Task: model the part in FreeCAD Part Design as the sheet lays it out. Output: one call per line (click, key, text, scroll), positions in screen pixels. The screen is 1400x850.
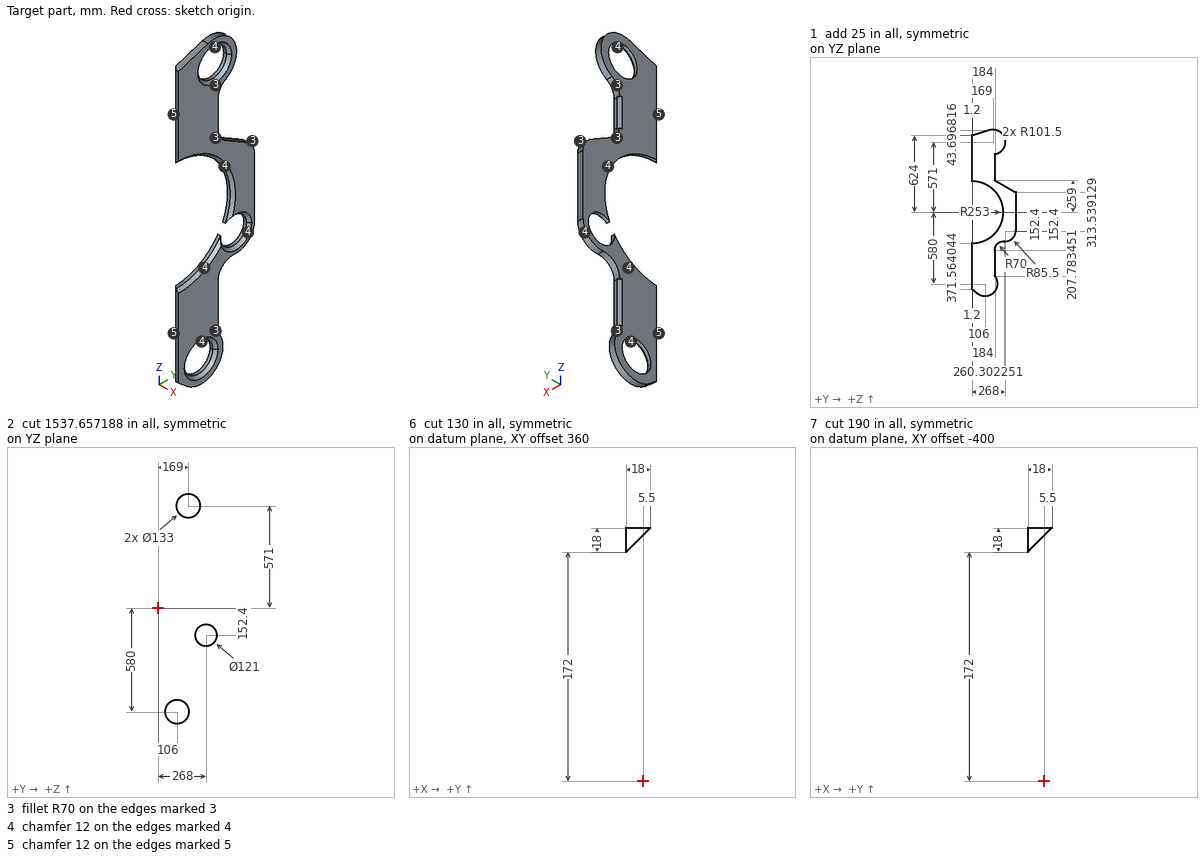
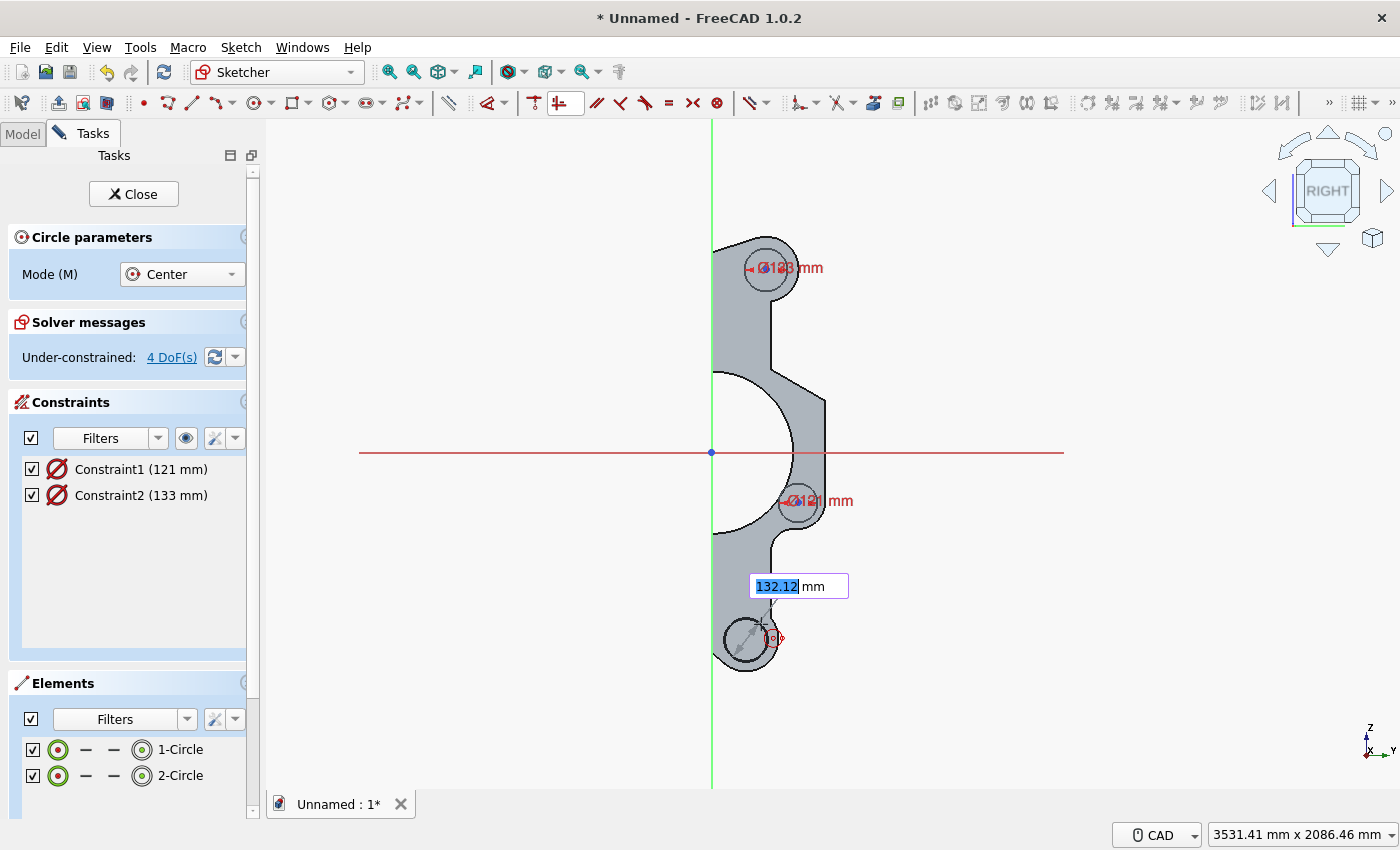
text(133)
key(Return)
key(Escape)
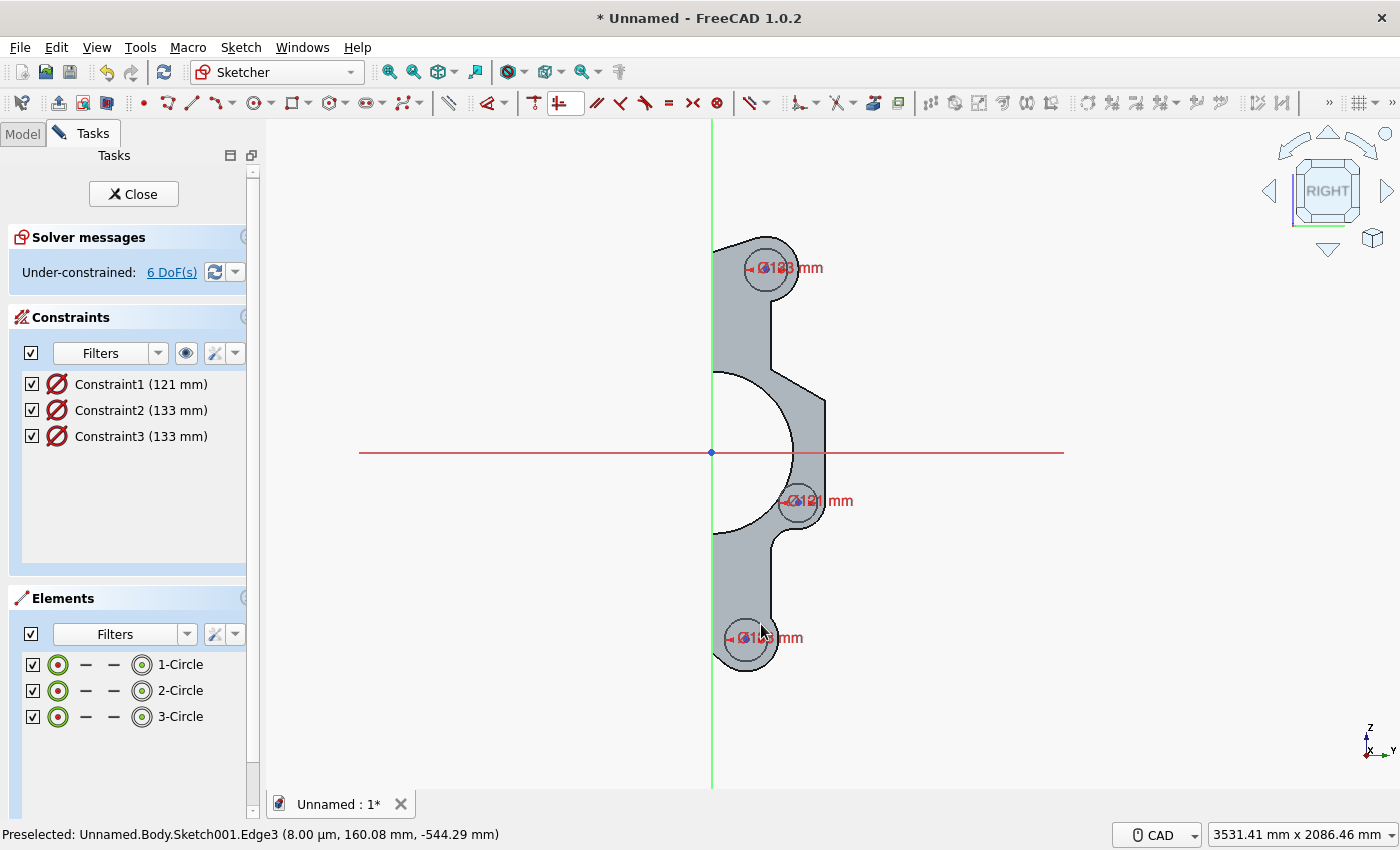
click(488, 104)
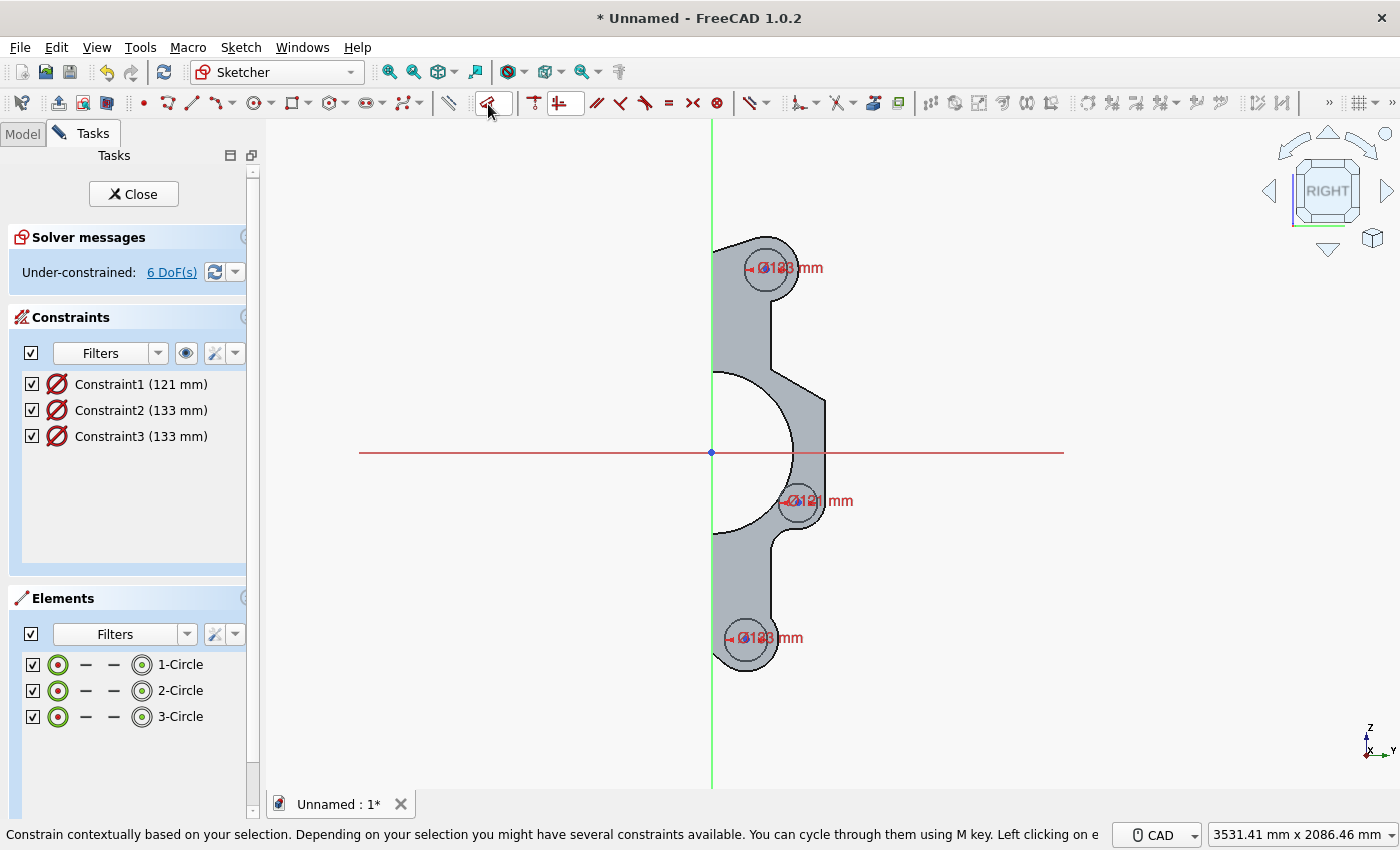
click(798, 503)
click(755, 537)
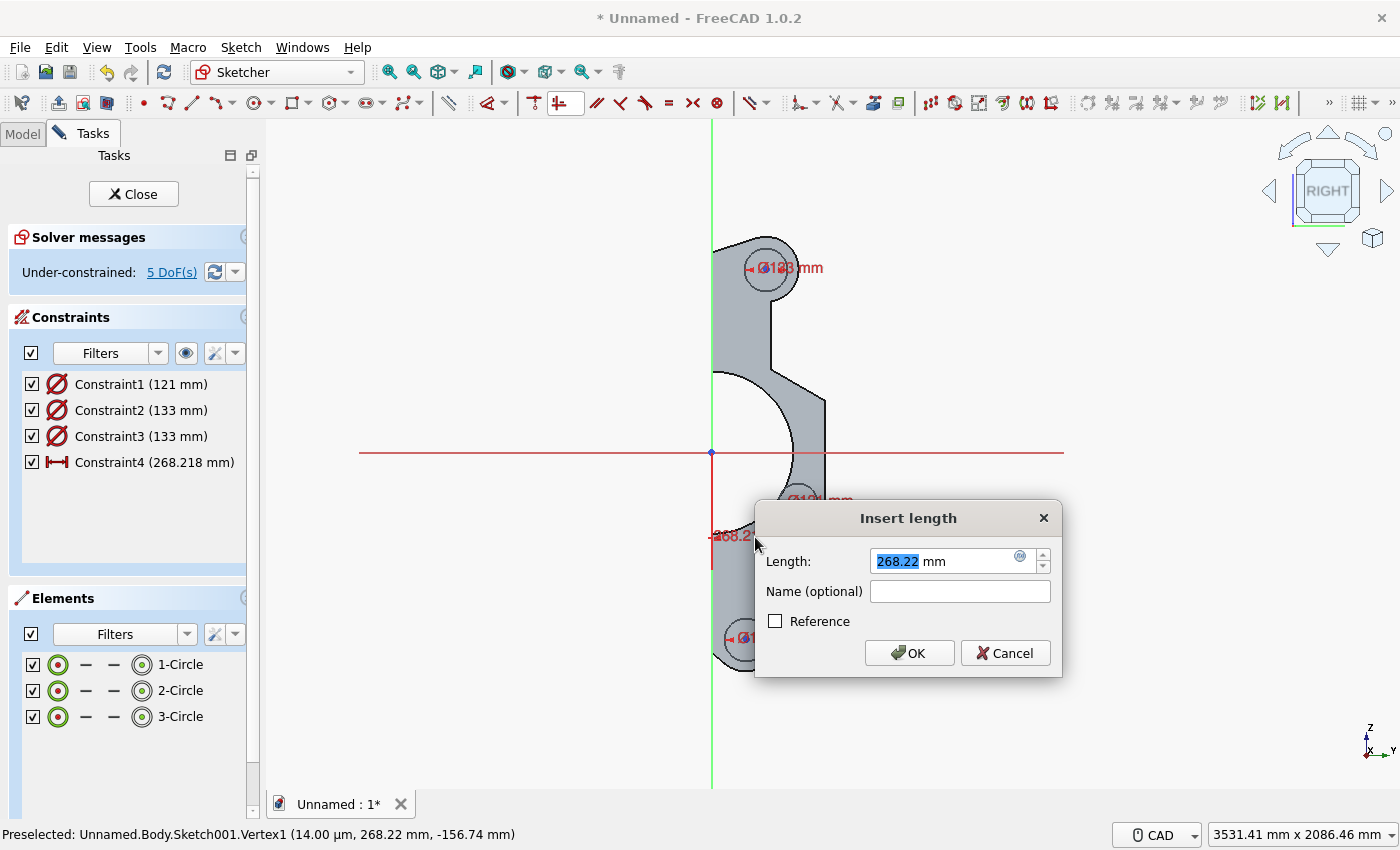
text(268)
key(Return)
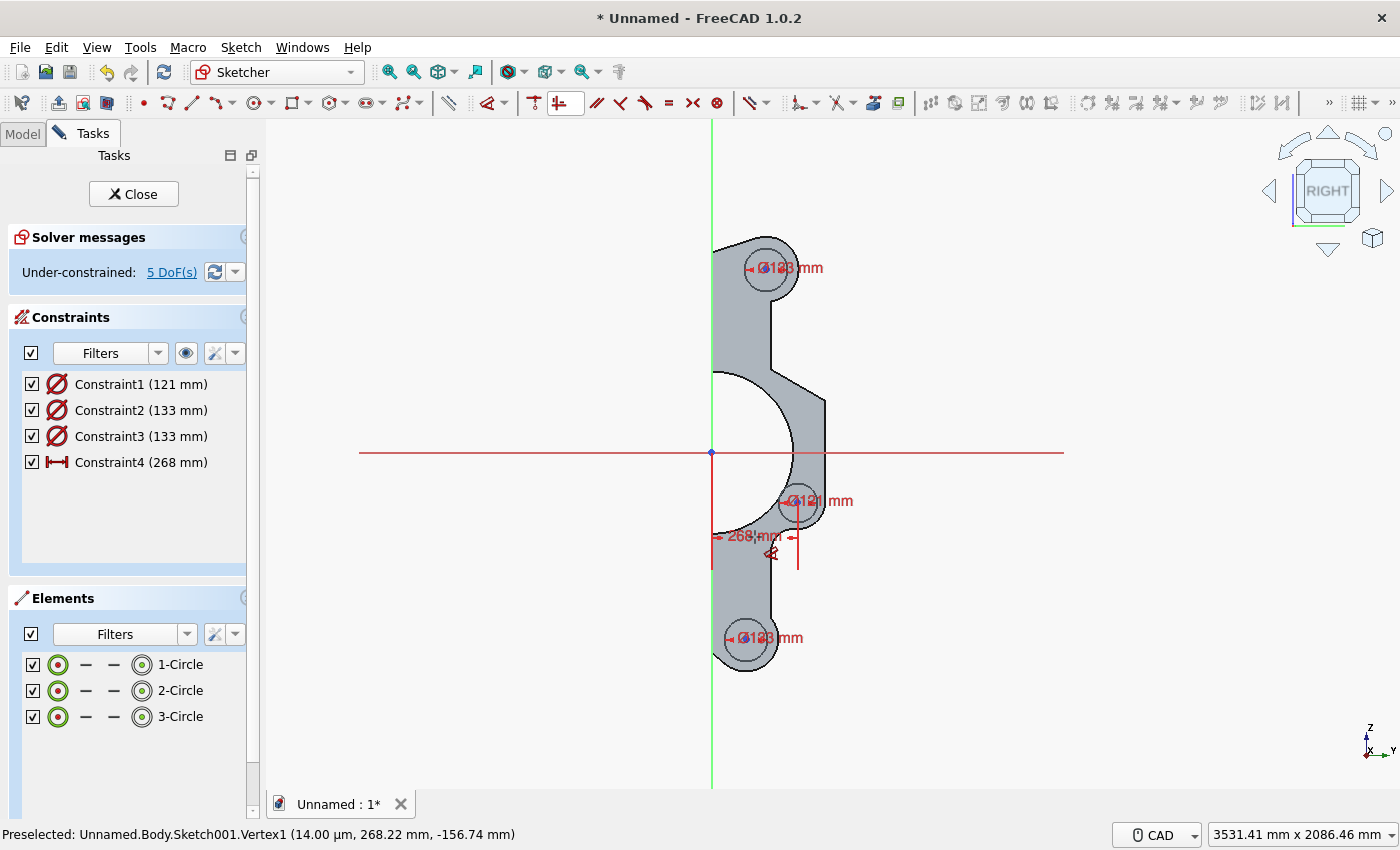
click(766, 270)
click(739, 236)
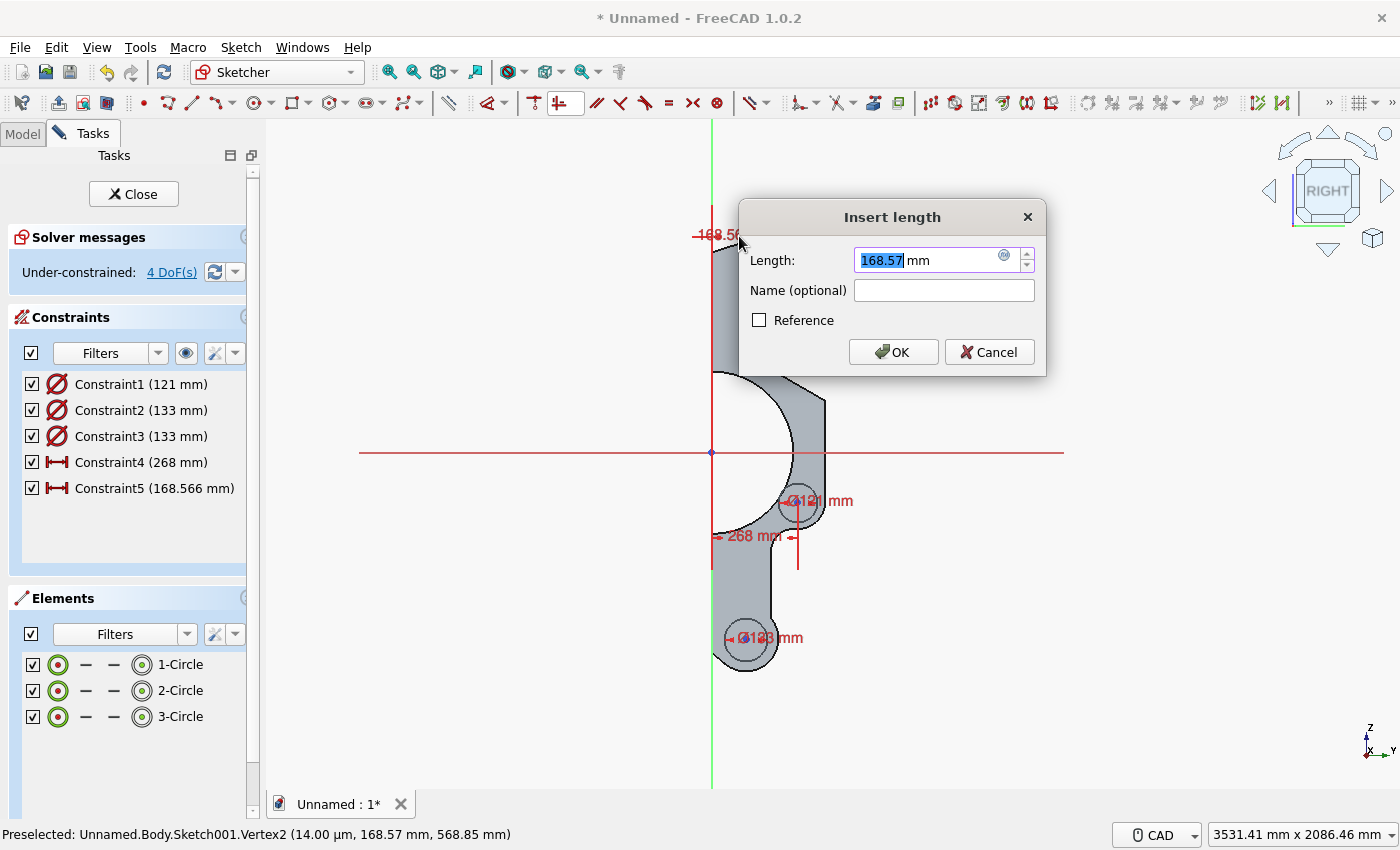
text(169)
key(Return)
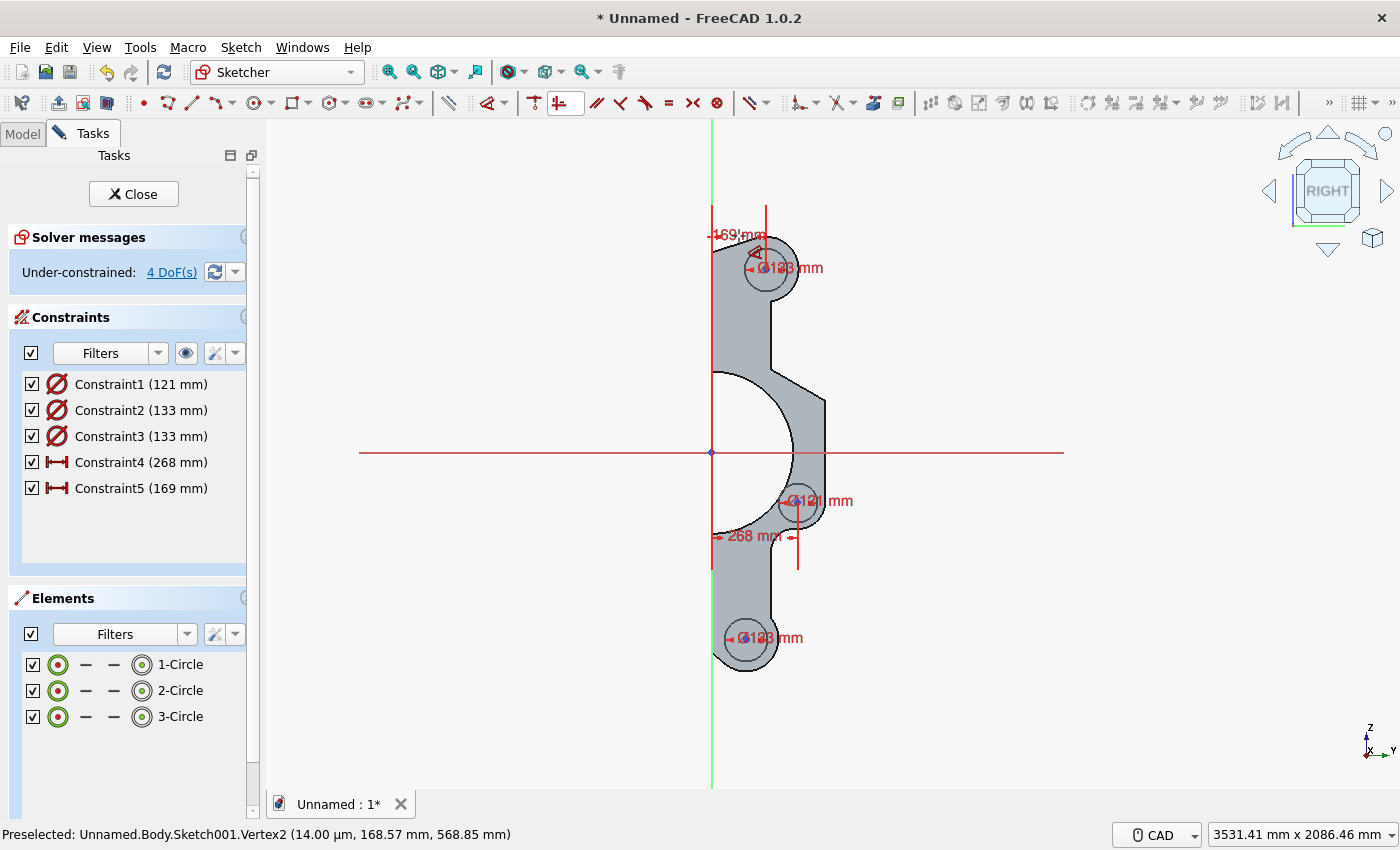
click(766, 270)
click(678, 361)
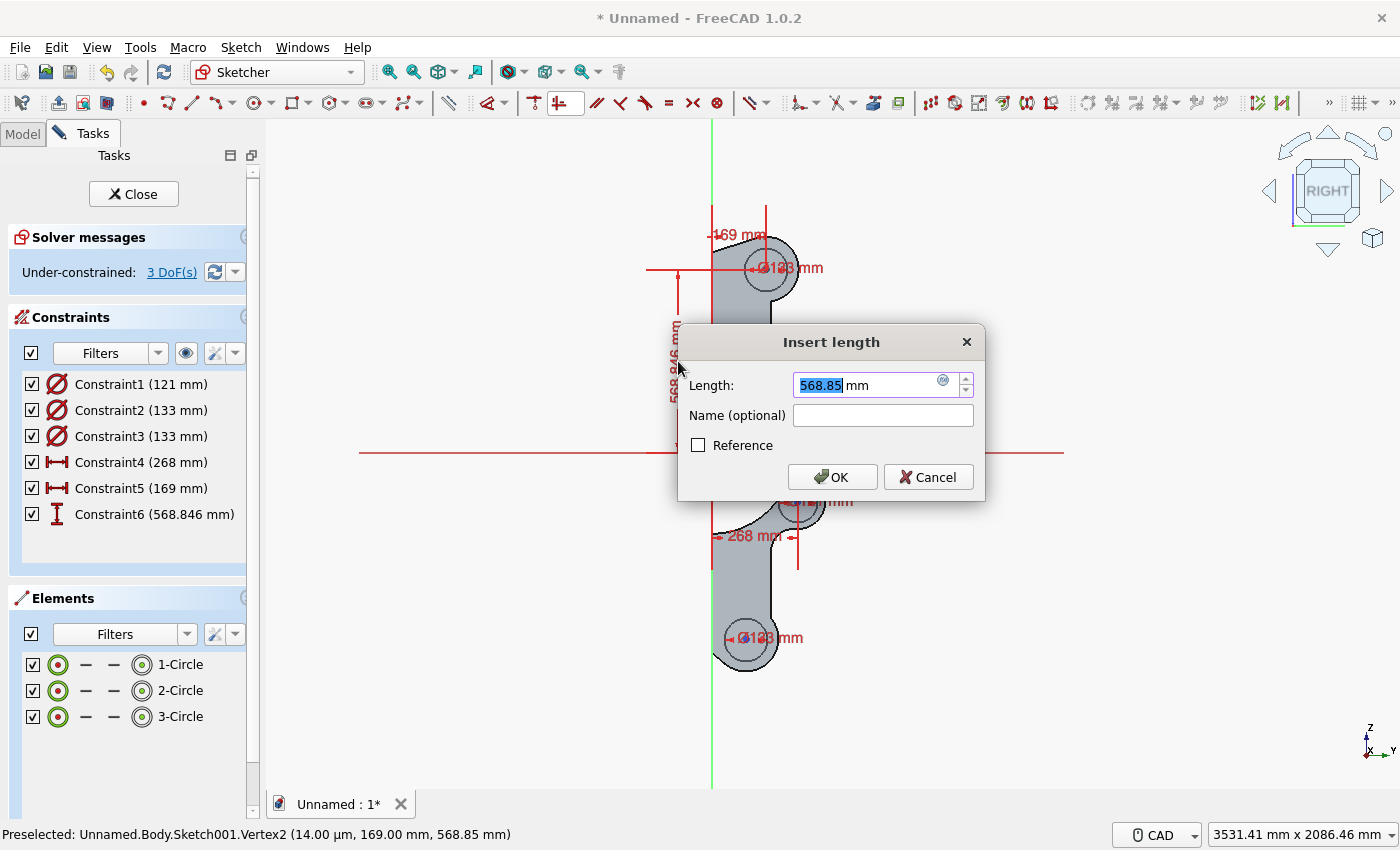
text(571)
key(Return)